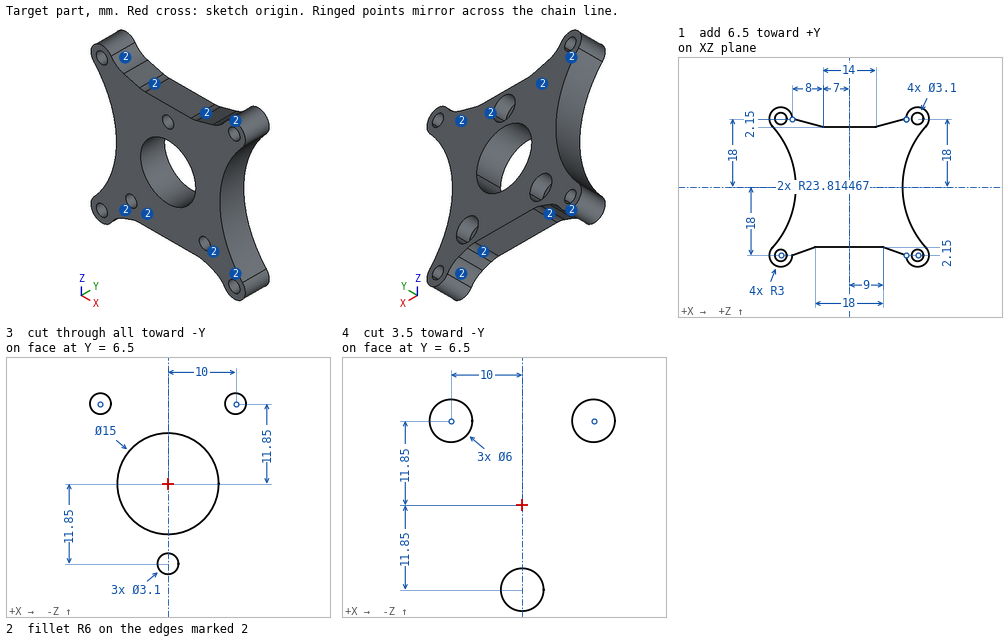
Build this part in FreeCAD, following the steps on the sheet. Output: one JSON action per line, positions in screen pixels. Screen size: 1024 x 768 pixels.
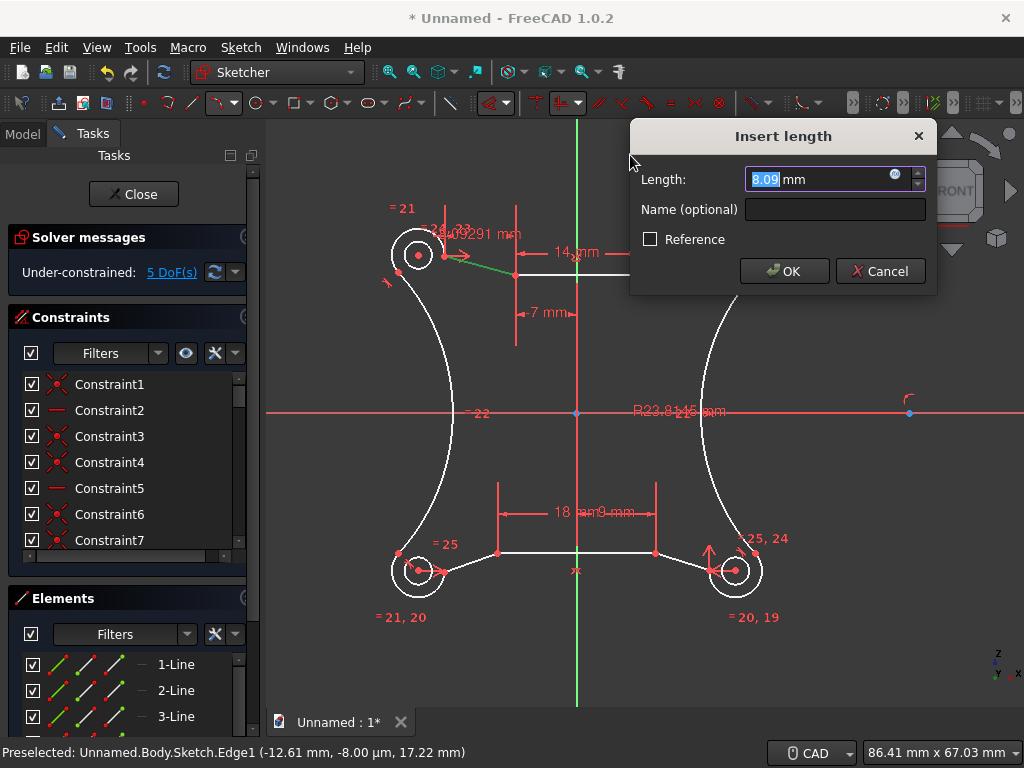
{"action": "type", "text": "8"}
{"action": "key", "text": "Return"}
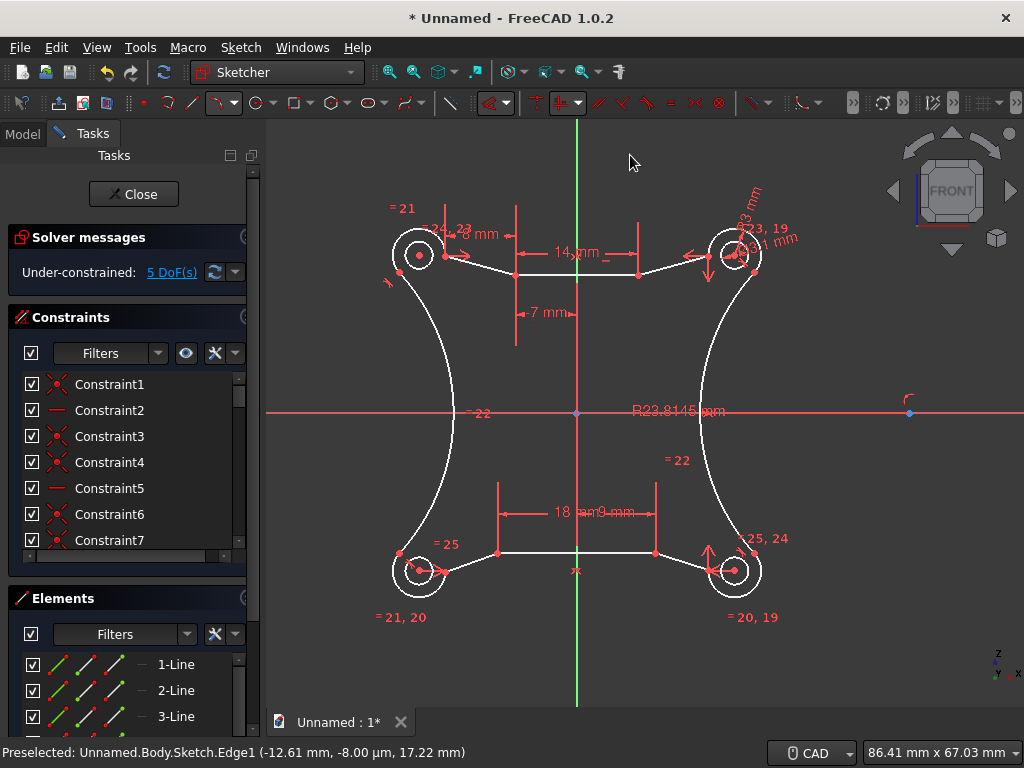
{"action": "left_click", "coordinate": [735, 255]}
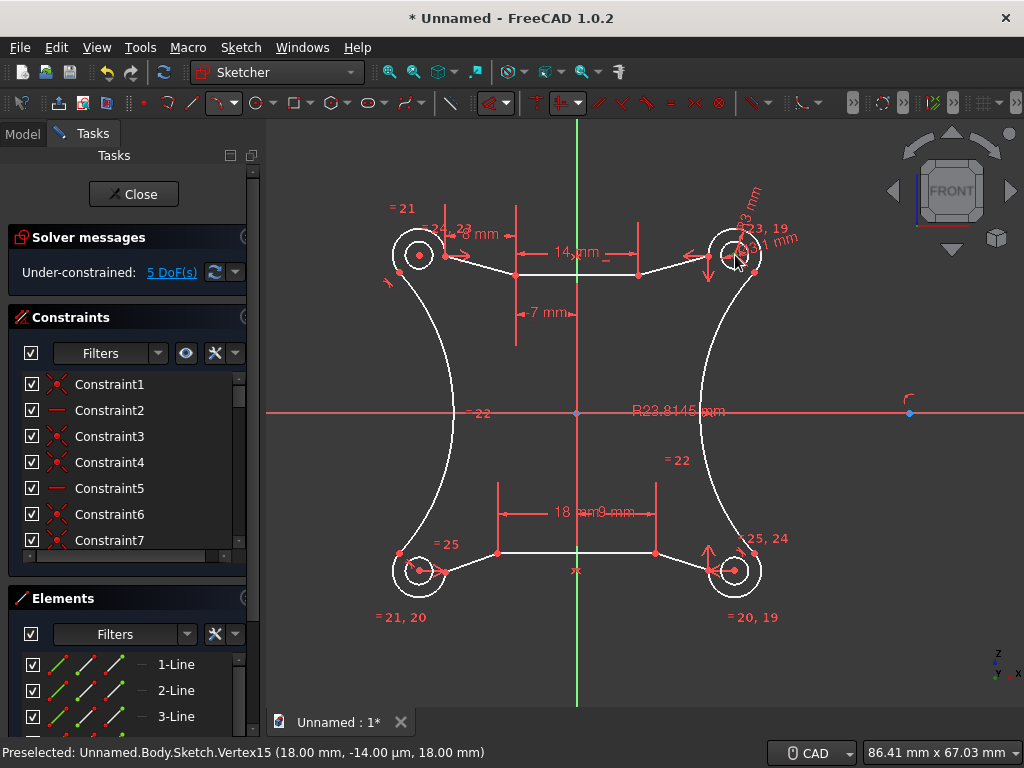
{"action": "left_click", "coordinate": [508, 104]}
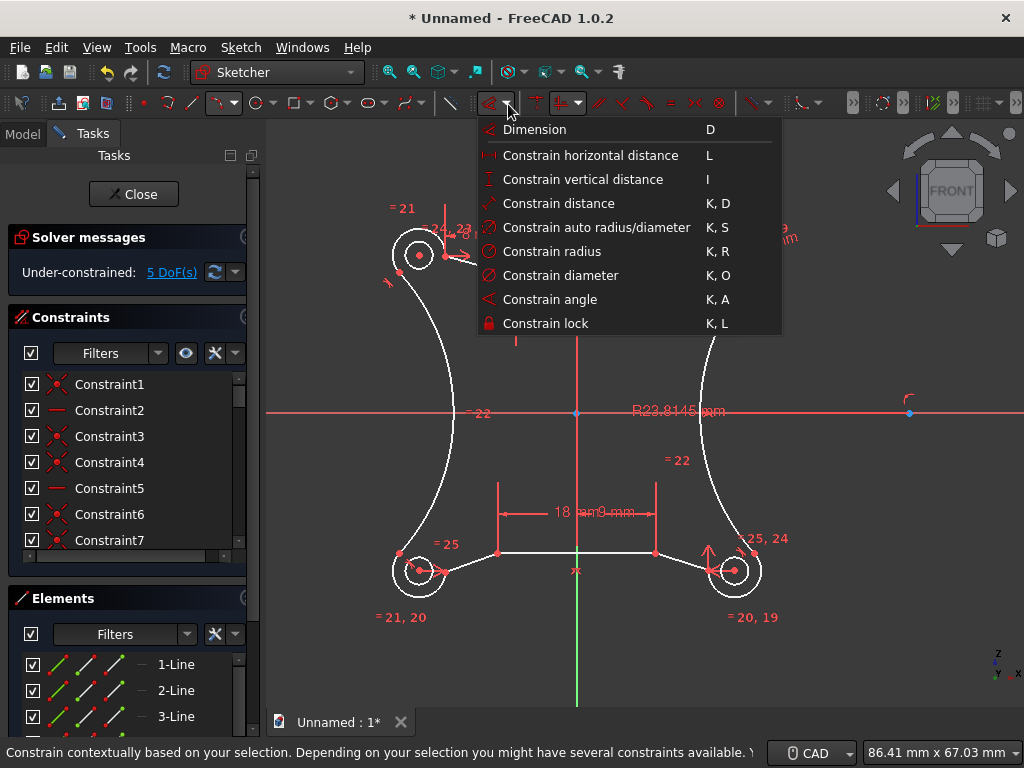
{"action": "left_click", "coordinate": [630, 179]}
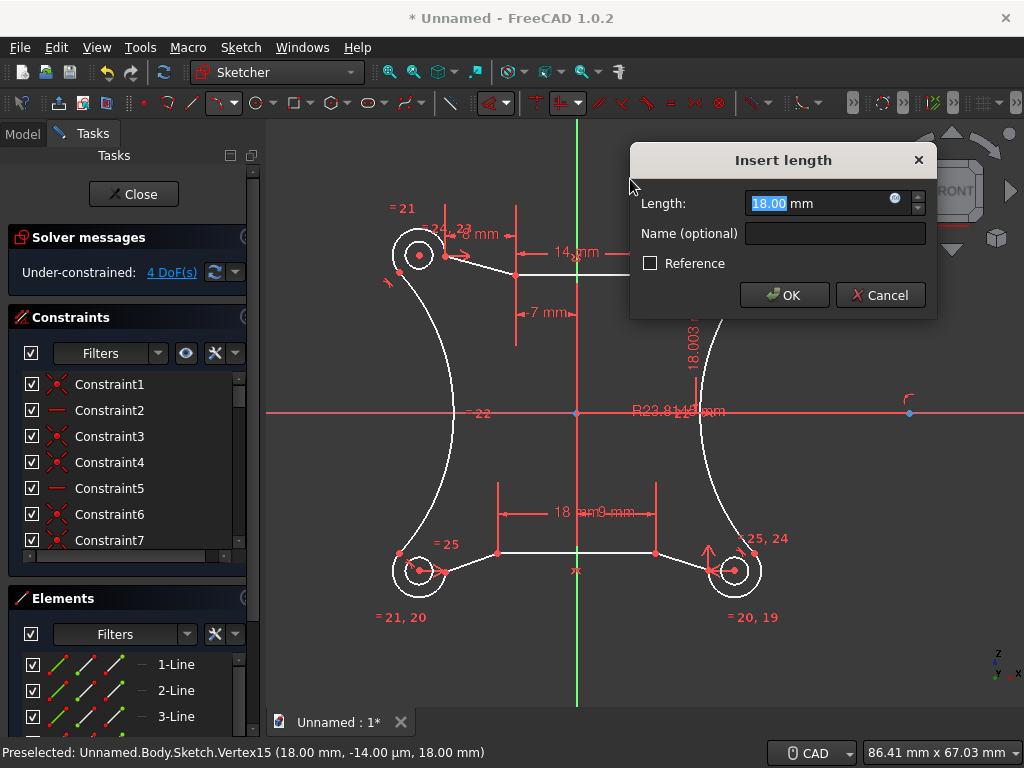
{"action": "type", "text": "18"}
{"action": "key", "text": "Return"}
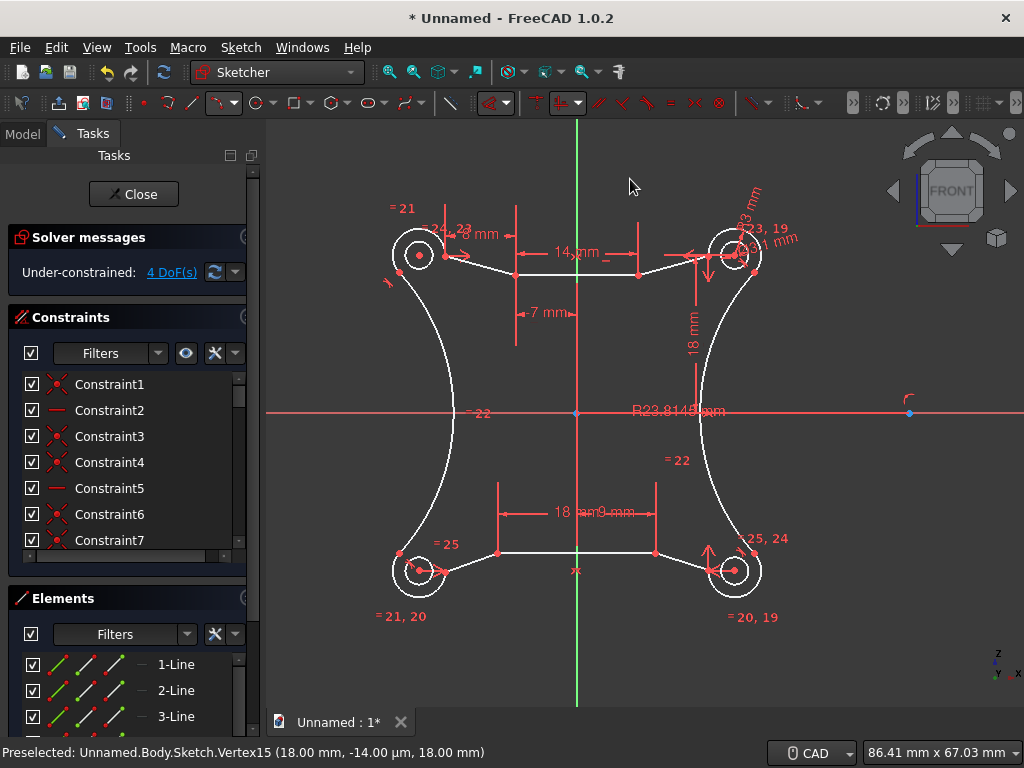
{"action": "left_click", "coordinate": [445, 256]}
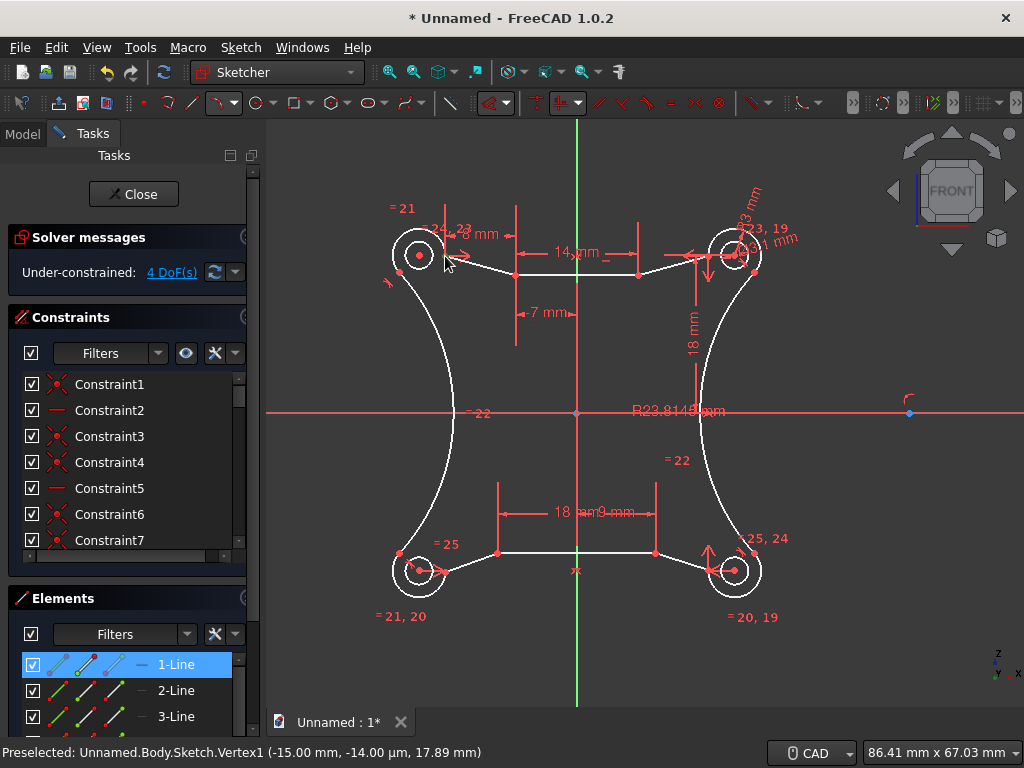
{"action": "key", "text": "i"}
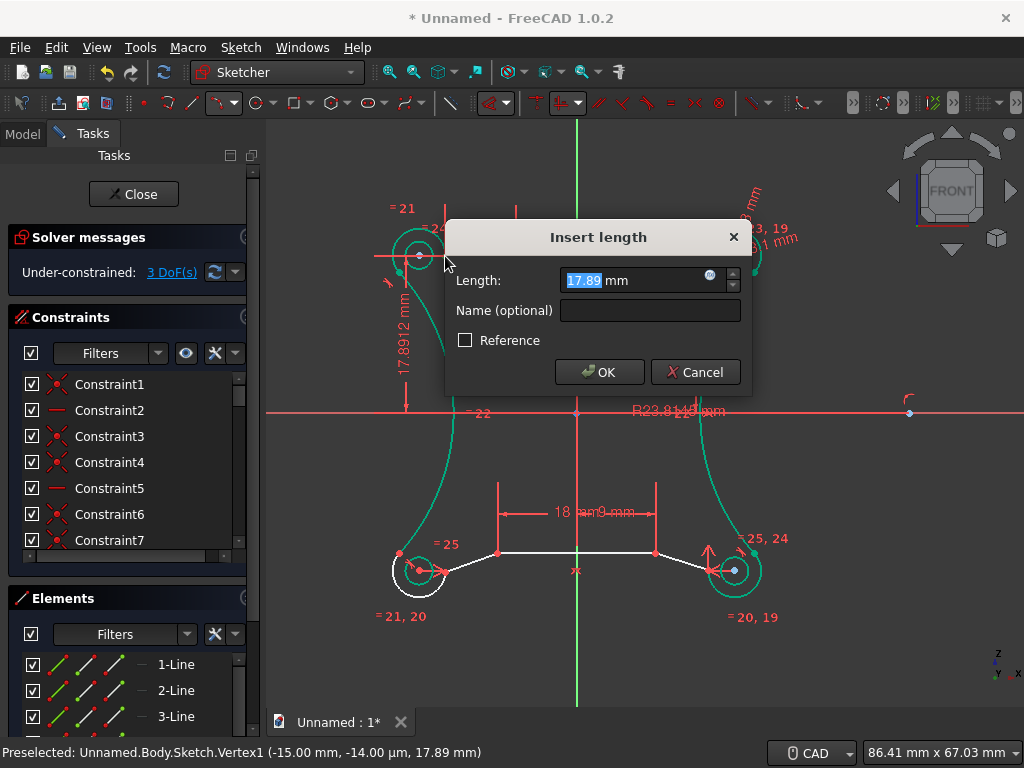
{"action": "type", "text": "18"}
{"action": "key", "text": "Return"}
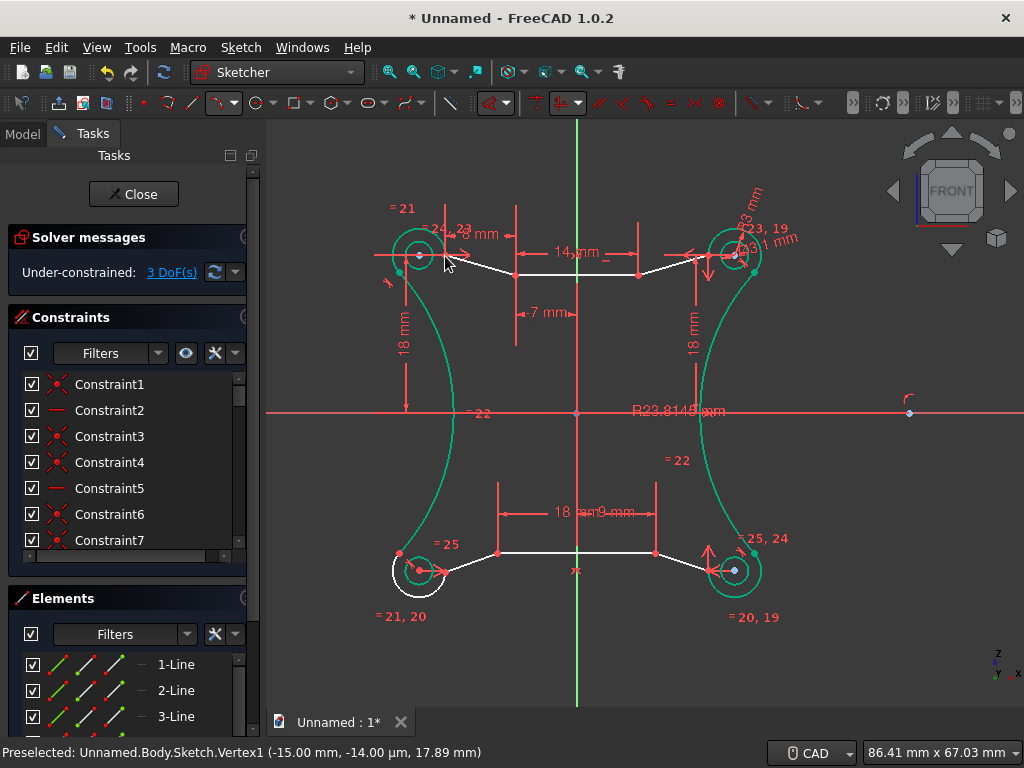
{"action": "left_click", "coordinate": [445, 572]}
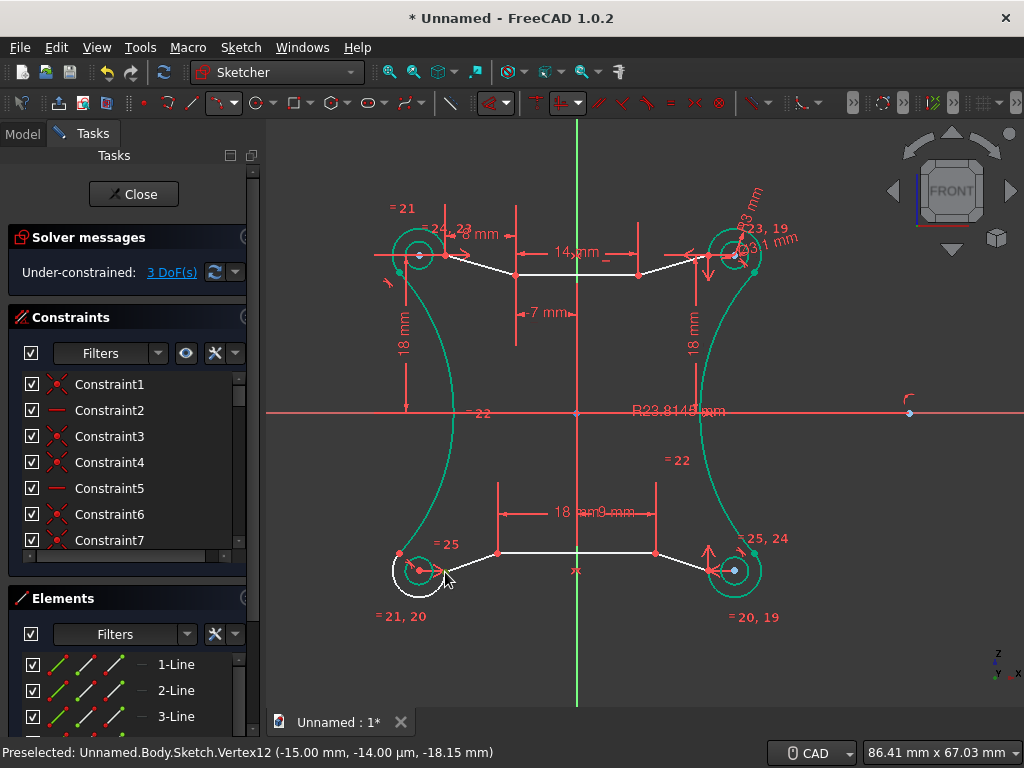
{"action": "left_click", "coordinate": [508, 104]}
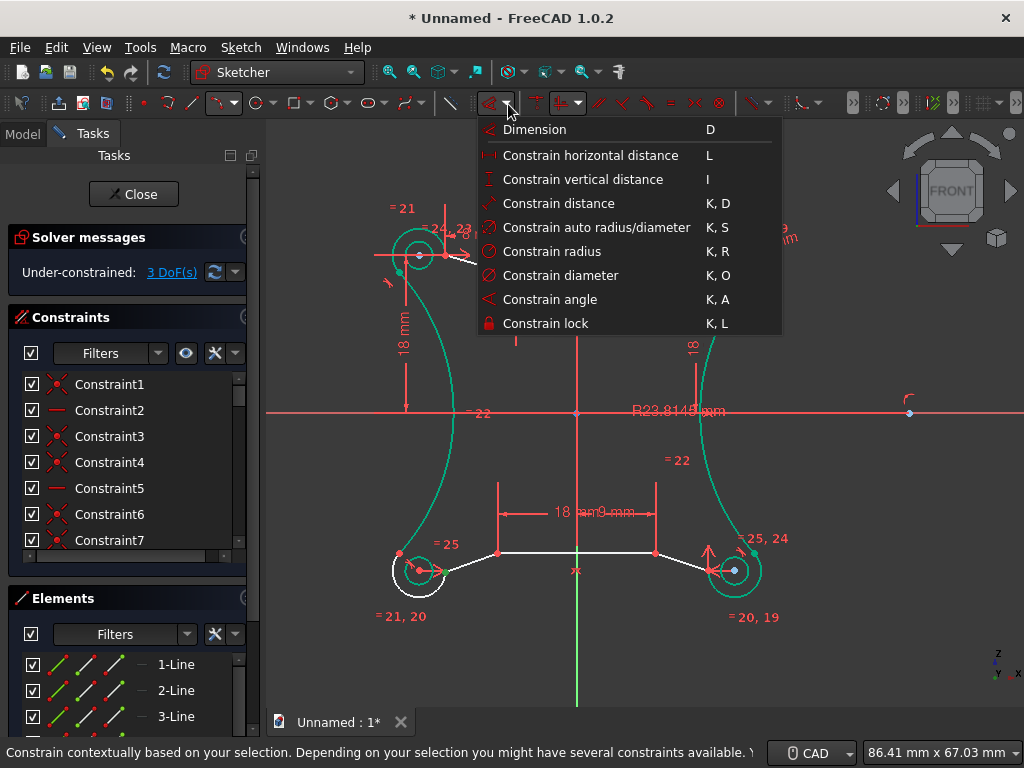
{"action": "left_click", "coordinate": [630, 179]}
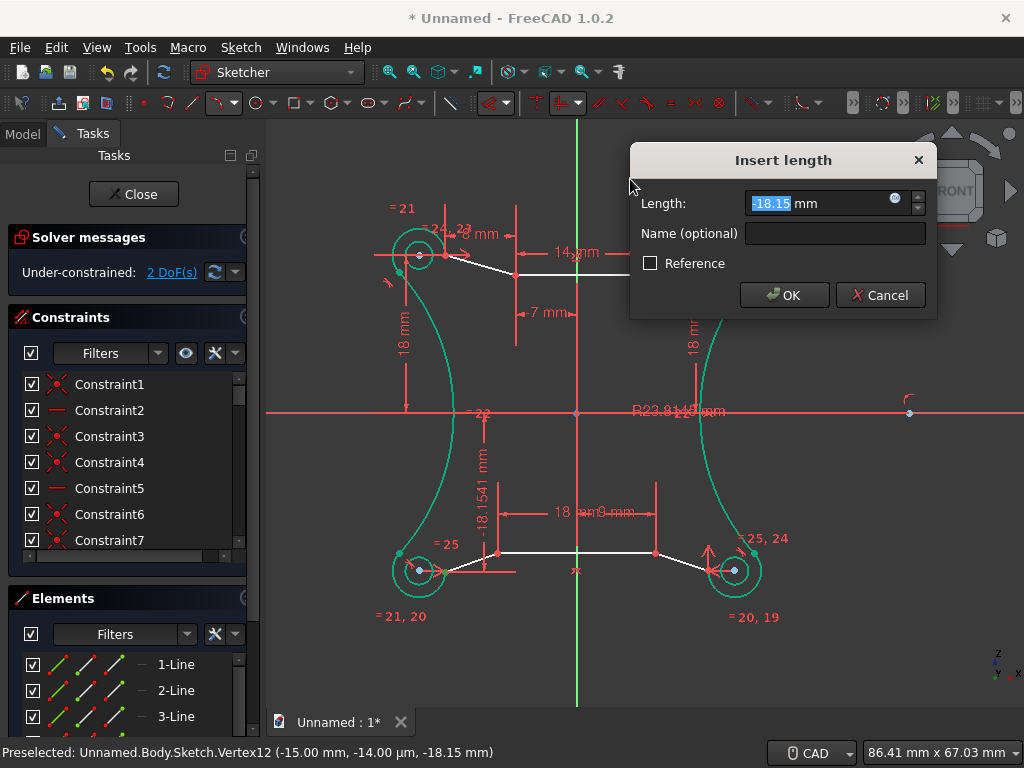
{"action": "type", "text": "-18"}
{"action": "key", "text": "Return"}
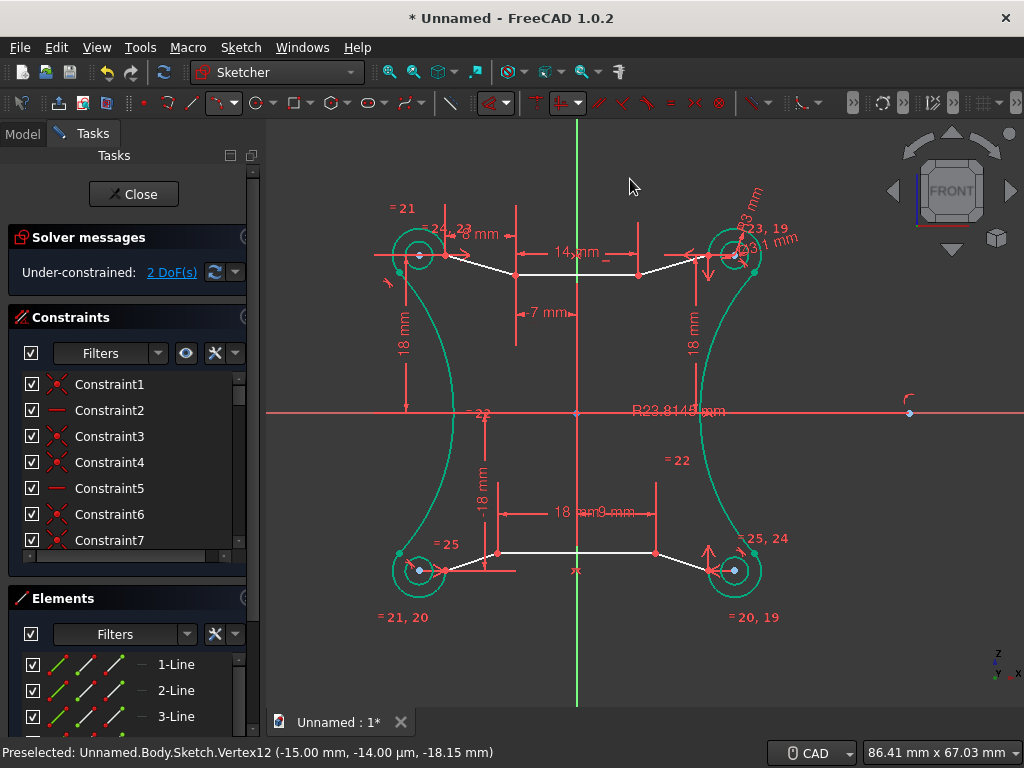
{"action": "scroll", "coordinate": [466, 261], "scroll_direction": "up", "scroll_amount": 4}